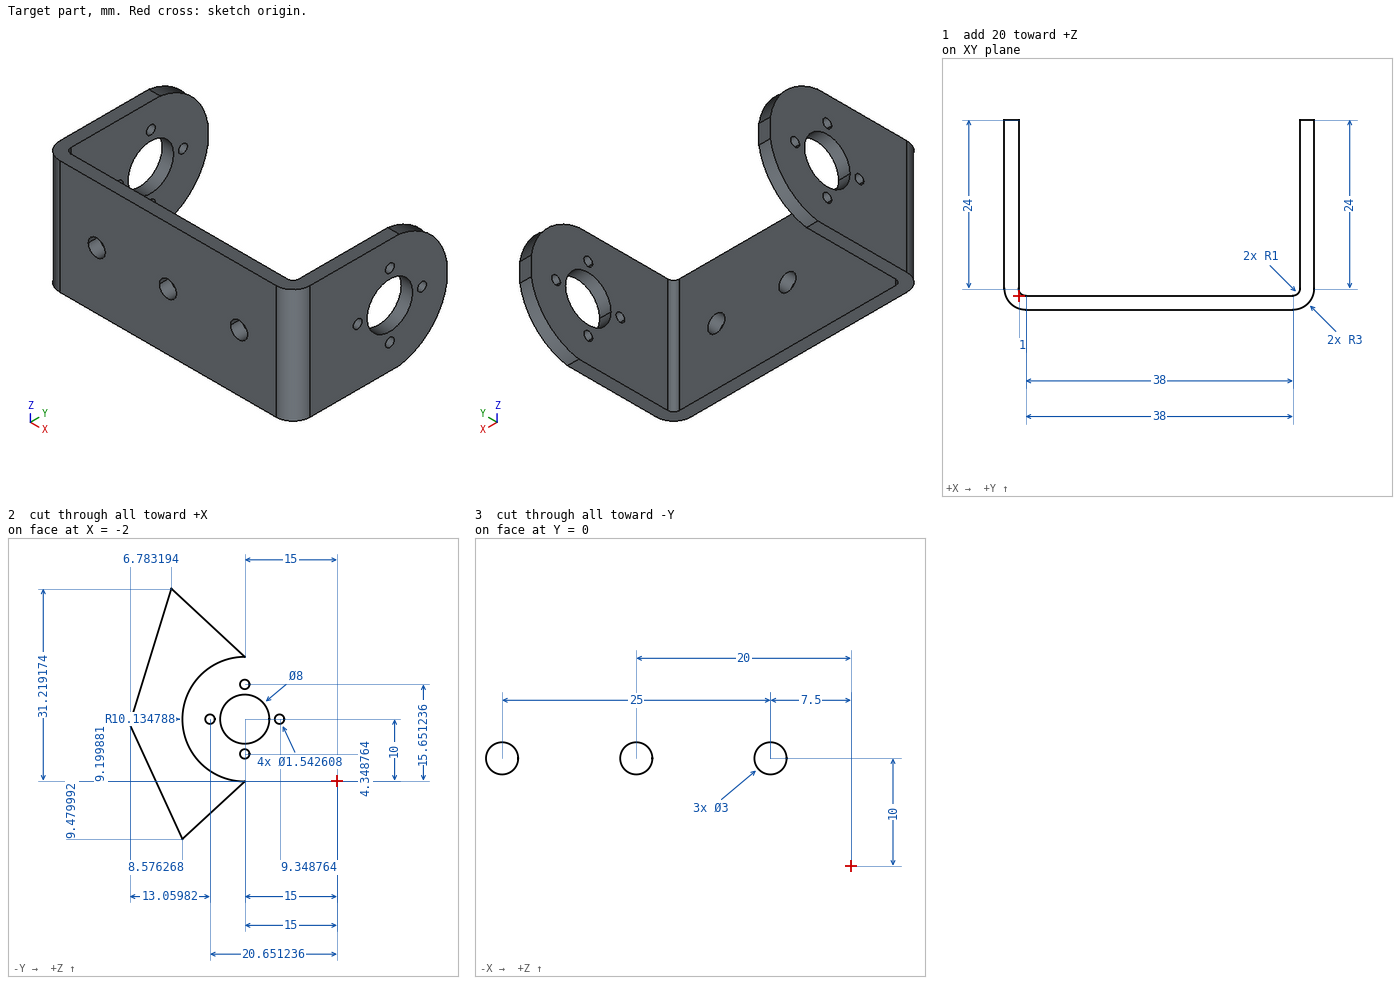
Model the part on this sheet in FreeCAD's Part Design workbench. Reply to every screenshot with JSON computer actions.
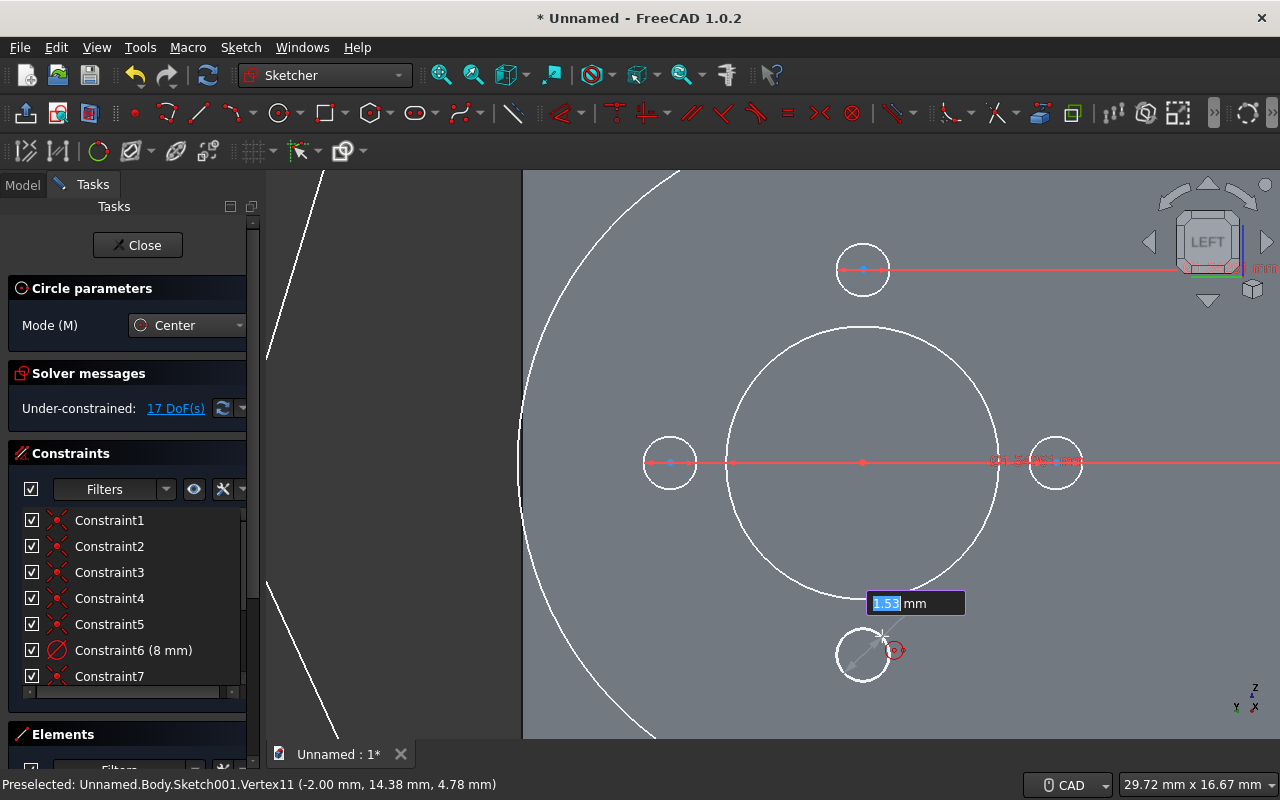
{"action": "type", "text": "1.542608"}
{"action": "key", "text": "Return"}
{"action": "key", "text": "Escape"}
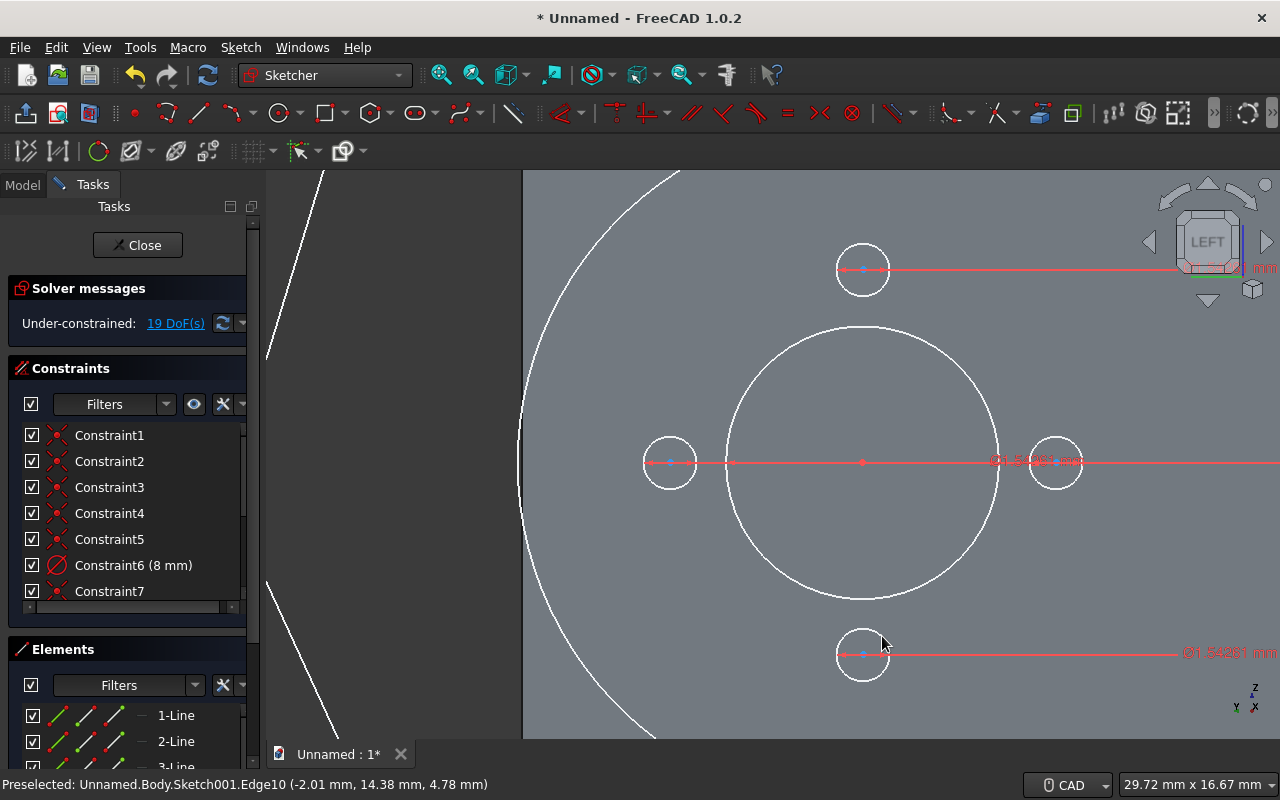
{"action": "left_click", "coordinate": [863, 463]}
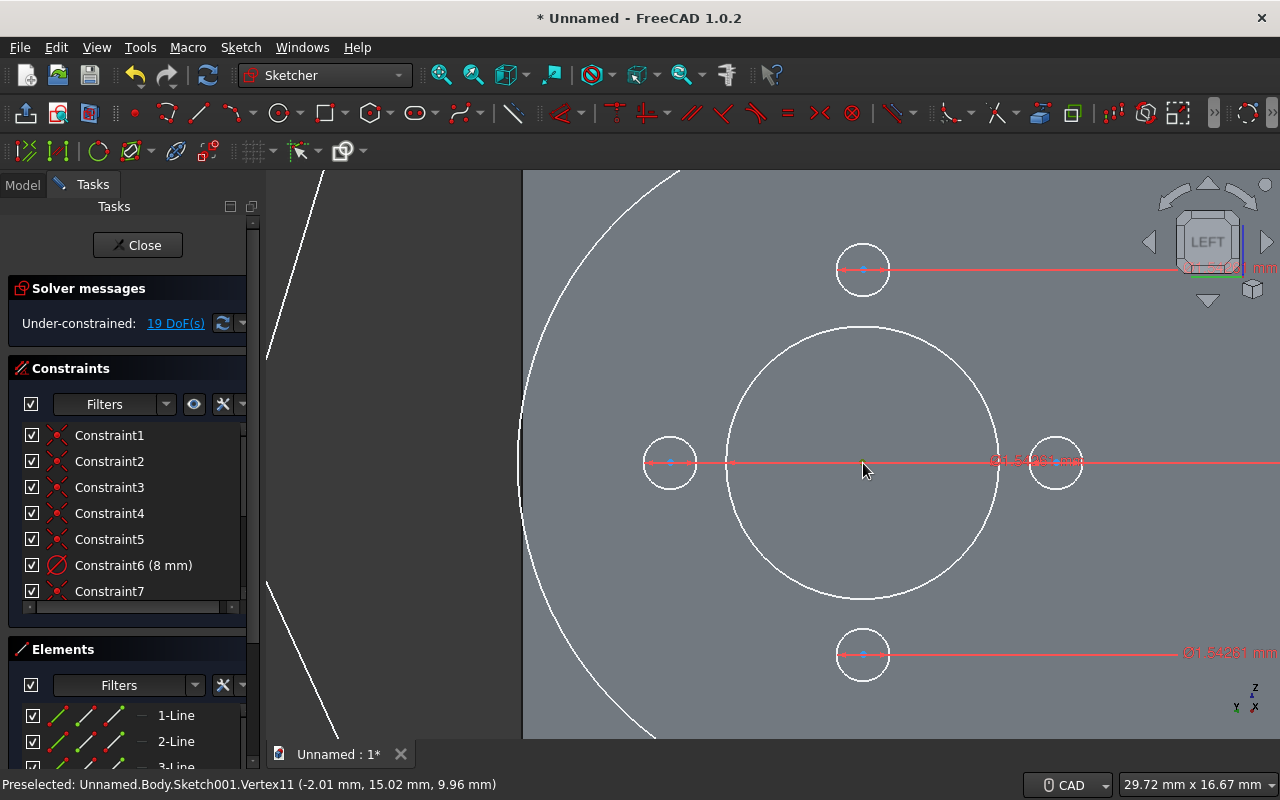
{"action": "left_click", "coordinate": [670, 463]}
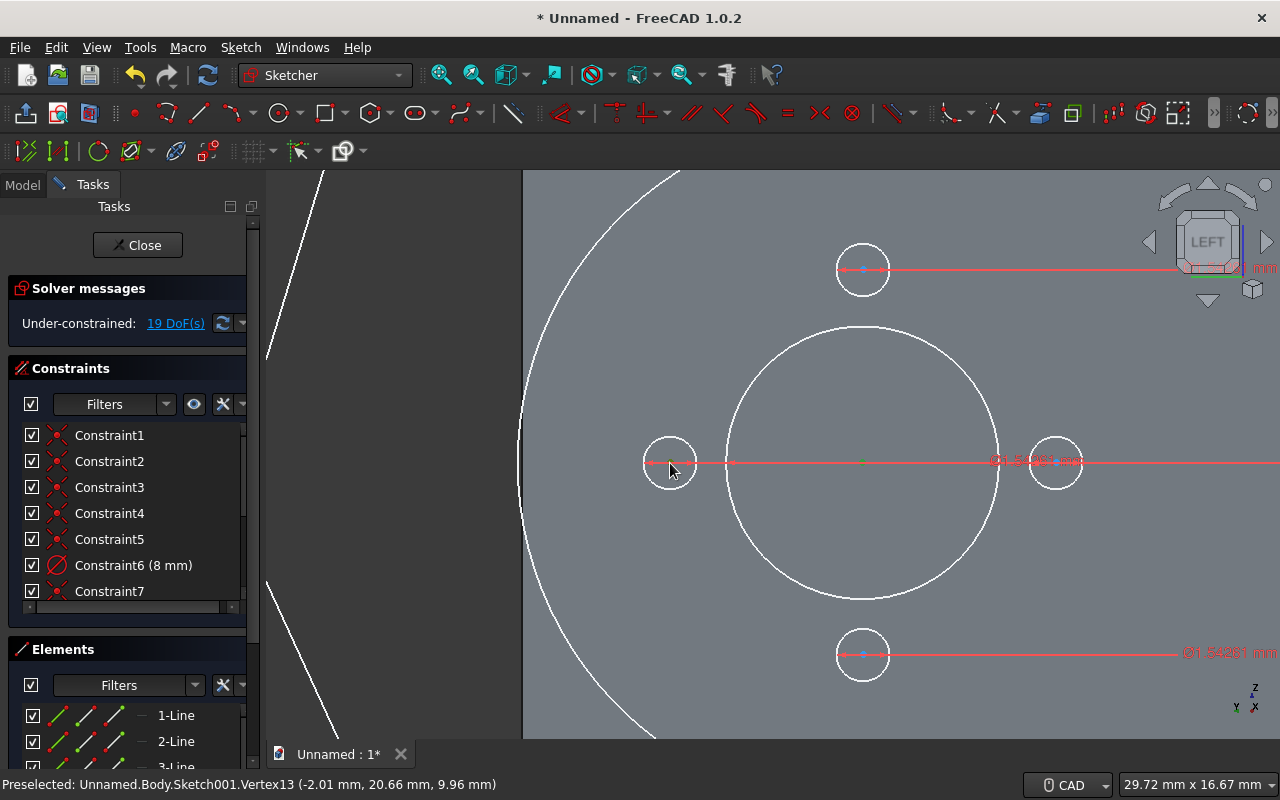
{"action": "left_click", "coordinate": [670, 114]}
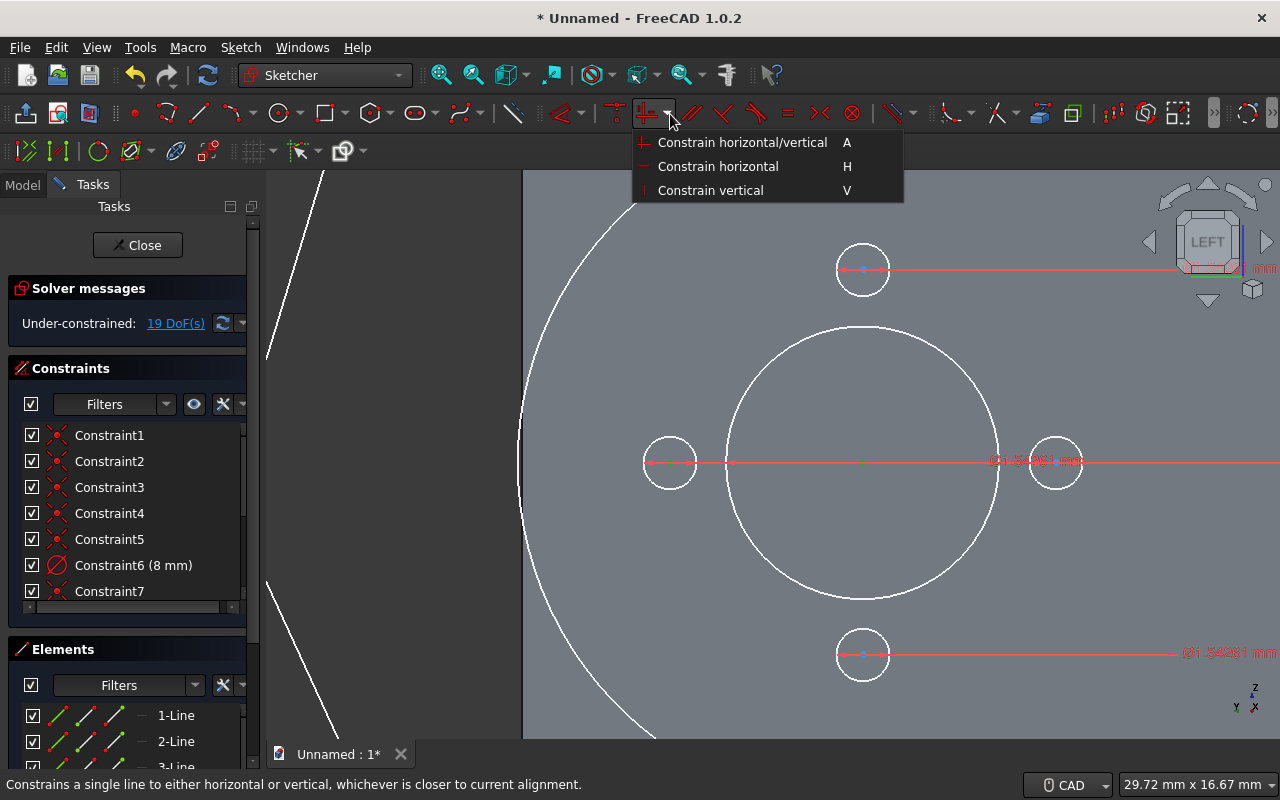
{"action": "left_click", "coordinate": [768, 166]}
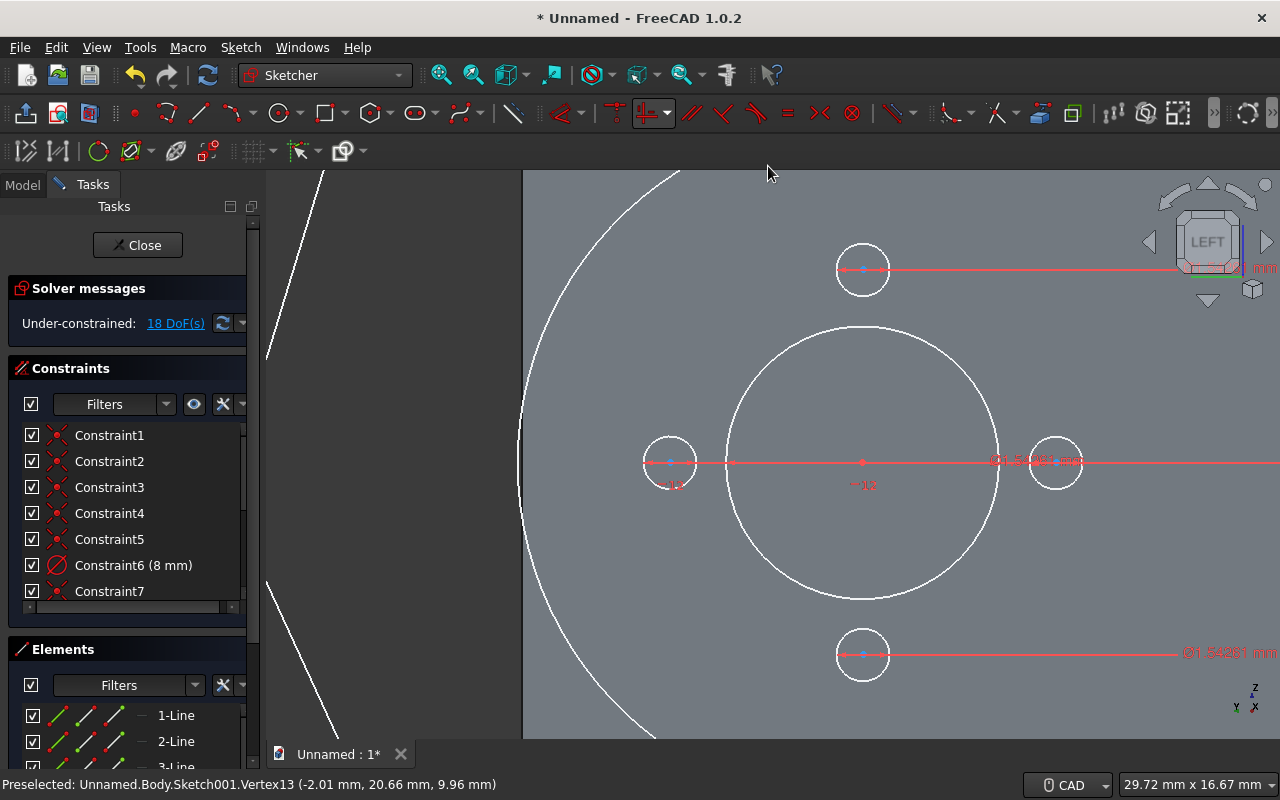
{"action": "left_click", "coordinate": [863, 463]}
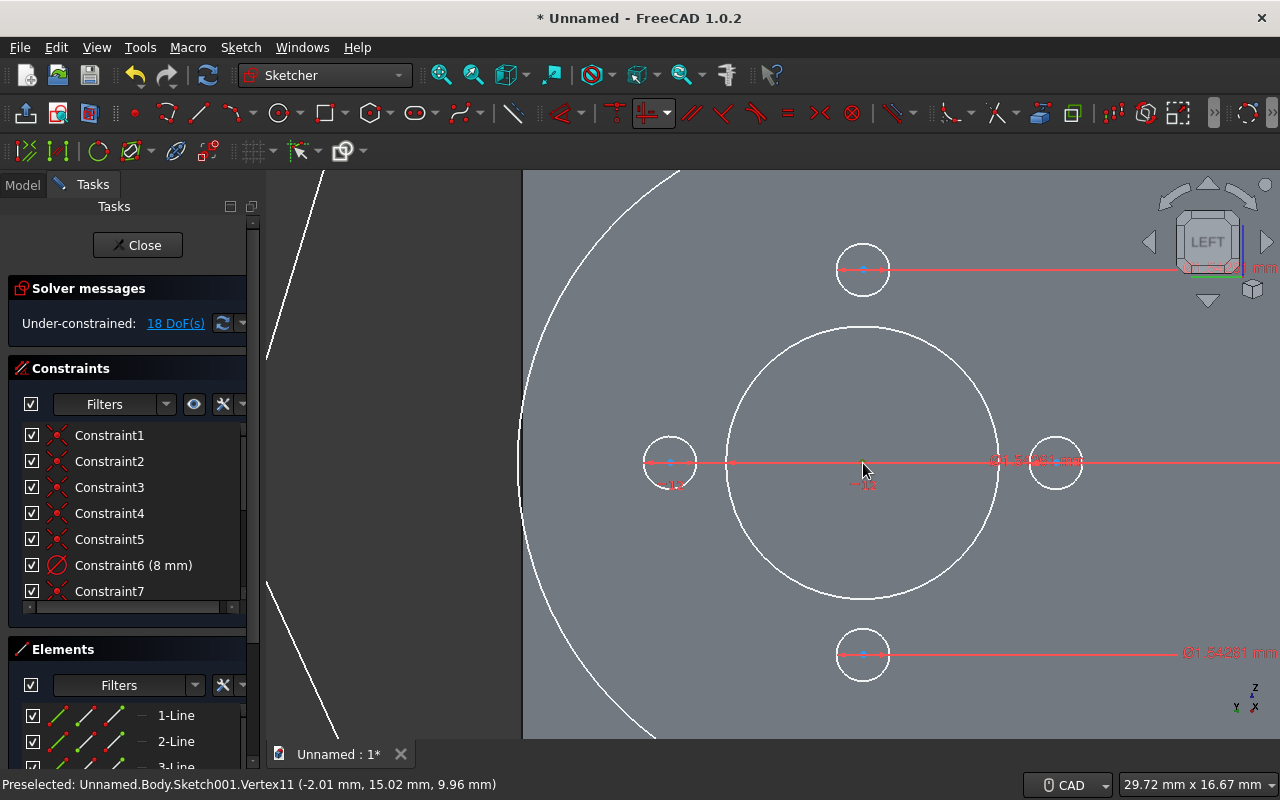
{"action": "left_click", "coordinate": [863, 270]}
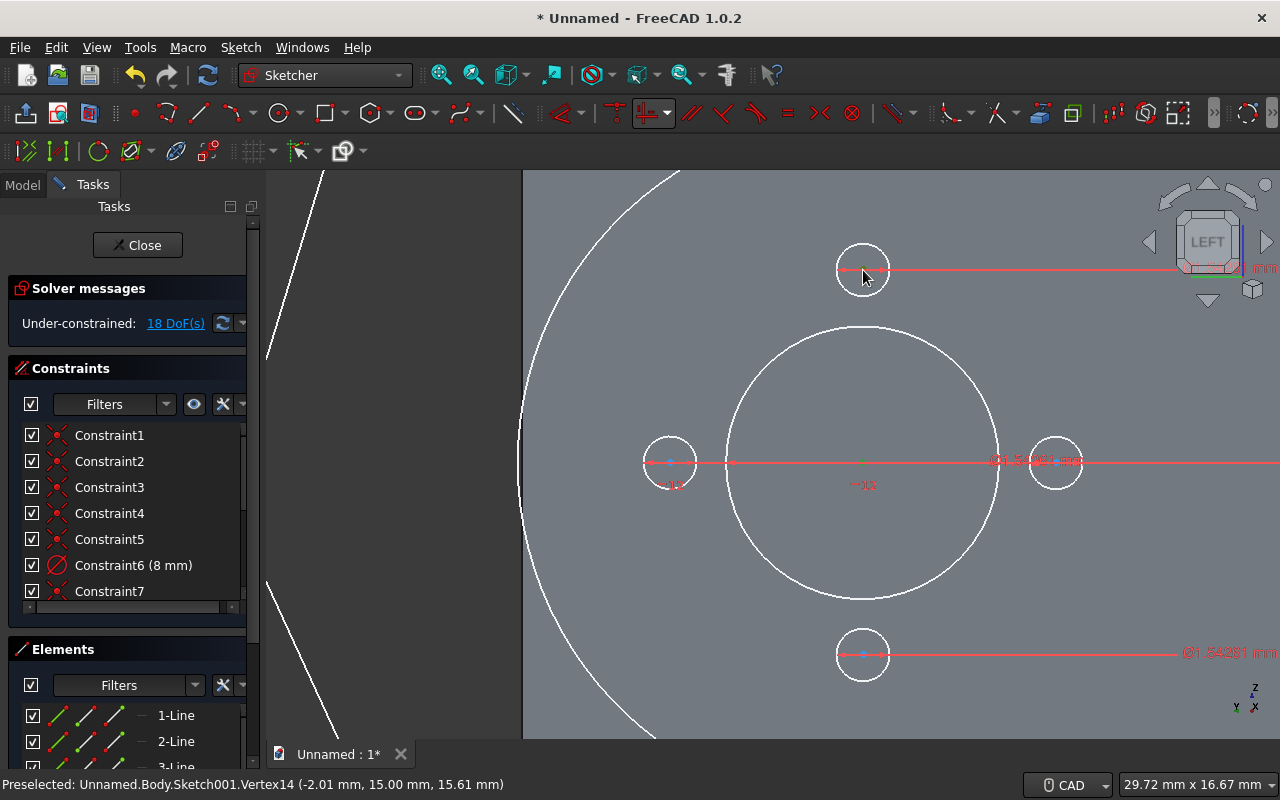
{"action": "key", "text": "v"}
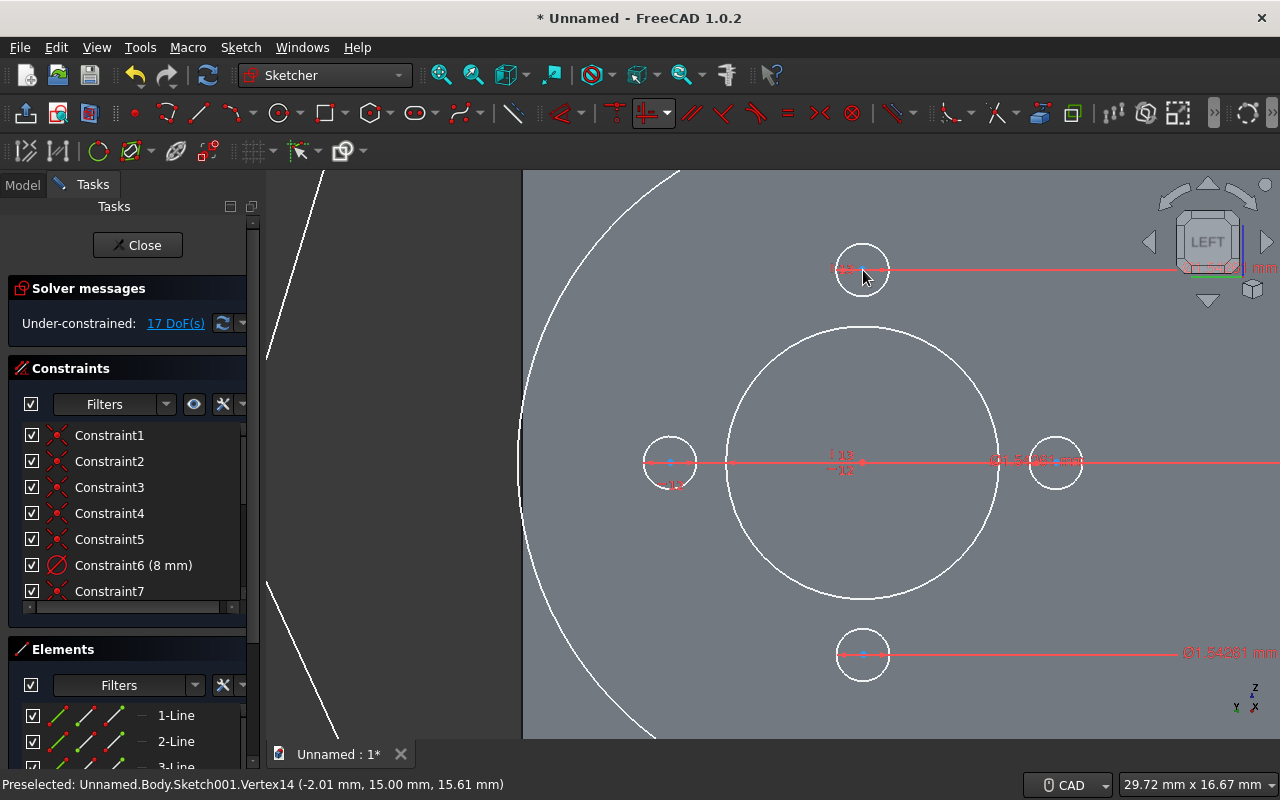
{"action": "left_click", "coordinate": [863, 463]}